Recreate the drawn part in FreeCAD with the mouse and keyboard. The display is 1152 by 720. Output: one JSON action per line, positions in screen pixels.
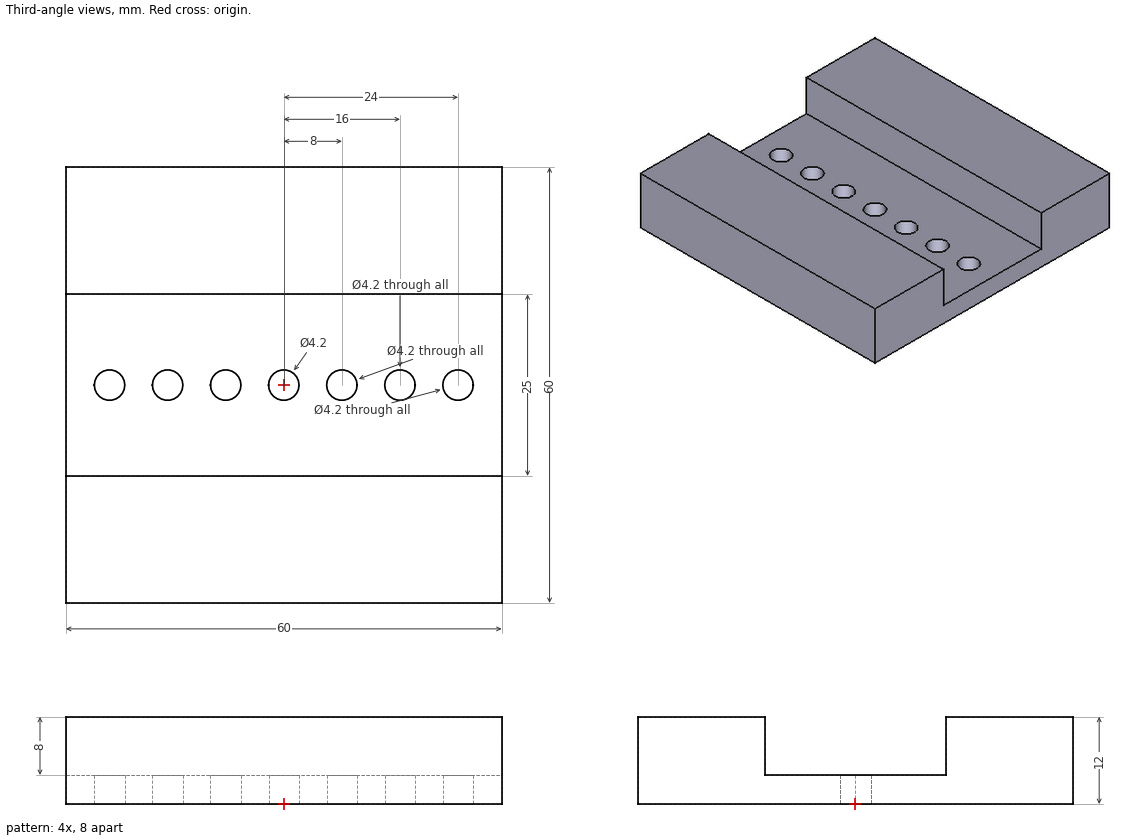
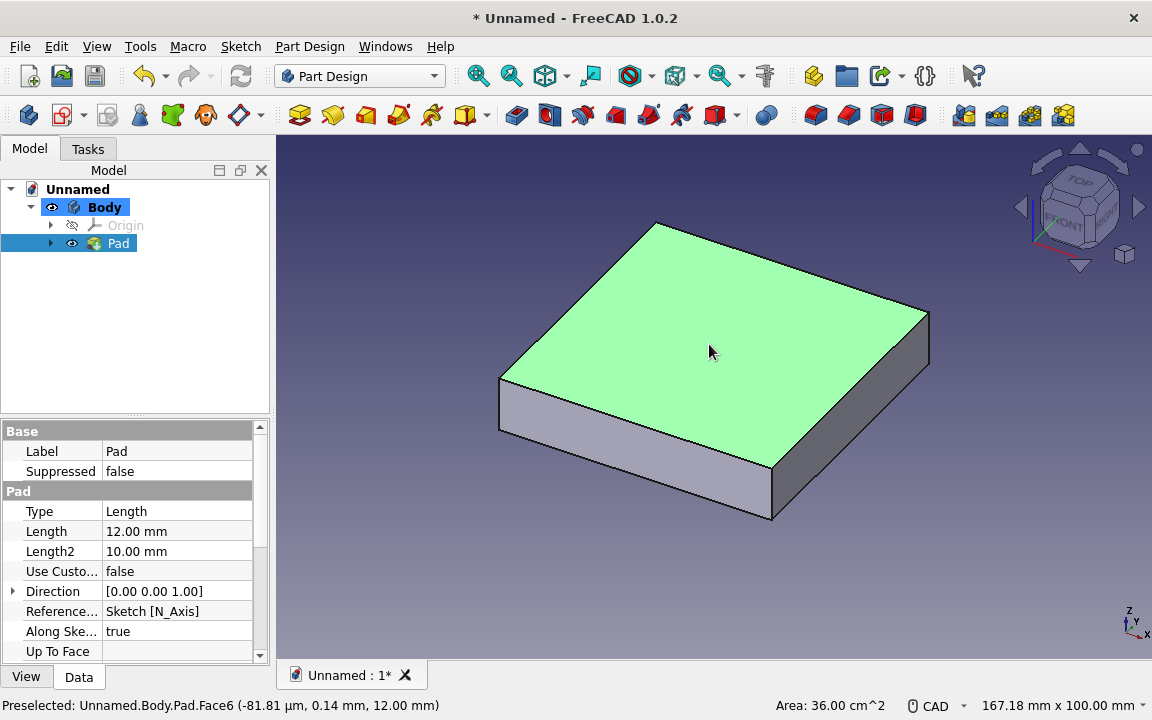
{"action": "left_click", "coordinate": [62, 116]}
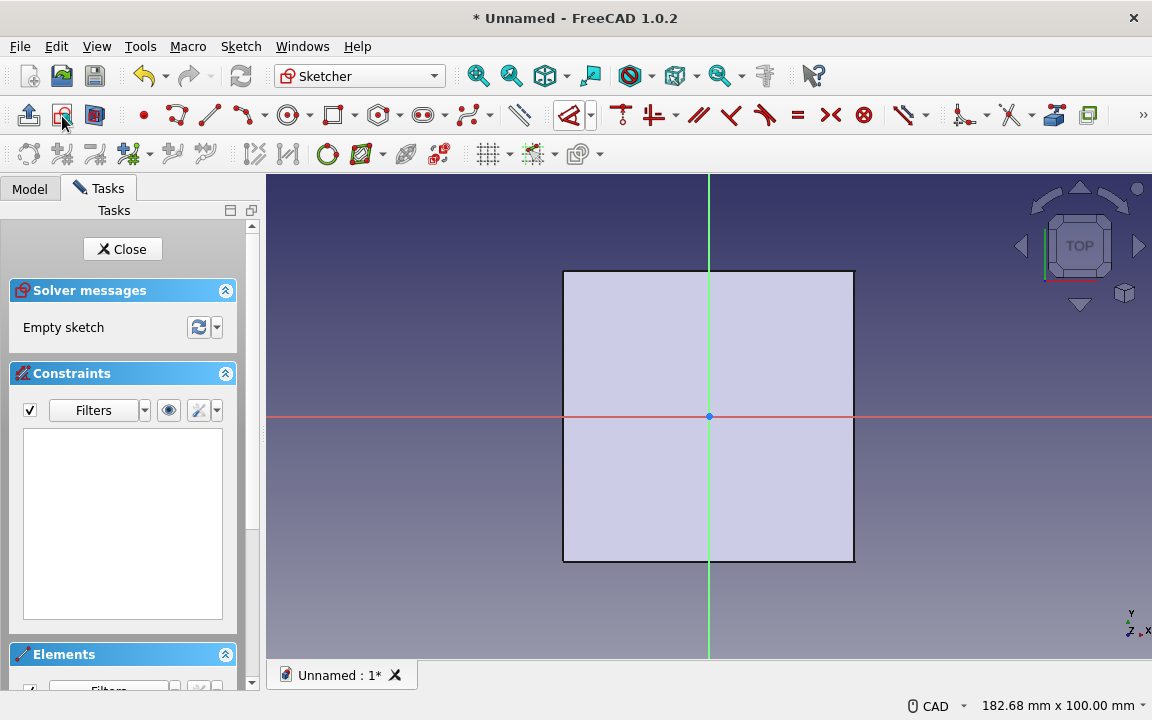
{"action": "scroll", "coordinate": [792, 416], "scroll_direction": "up", "scroll_amount": 3}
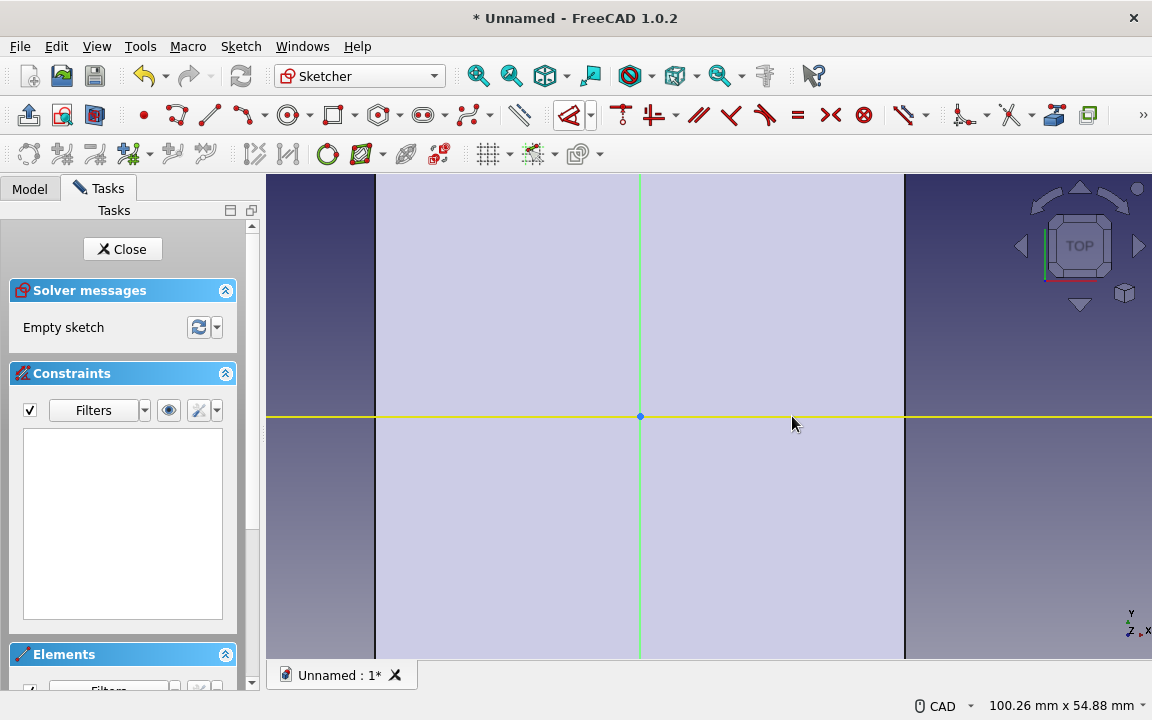
{"action": "left_click", "coordinate": [354, 116]}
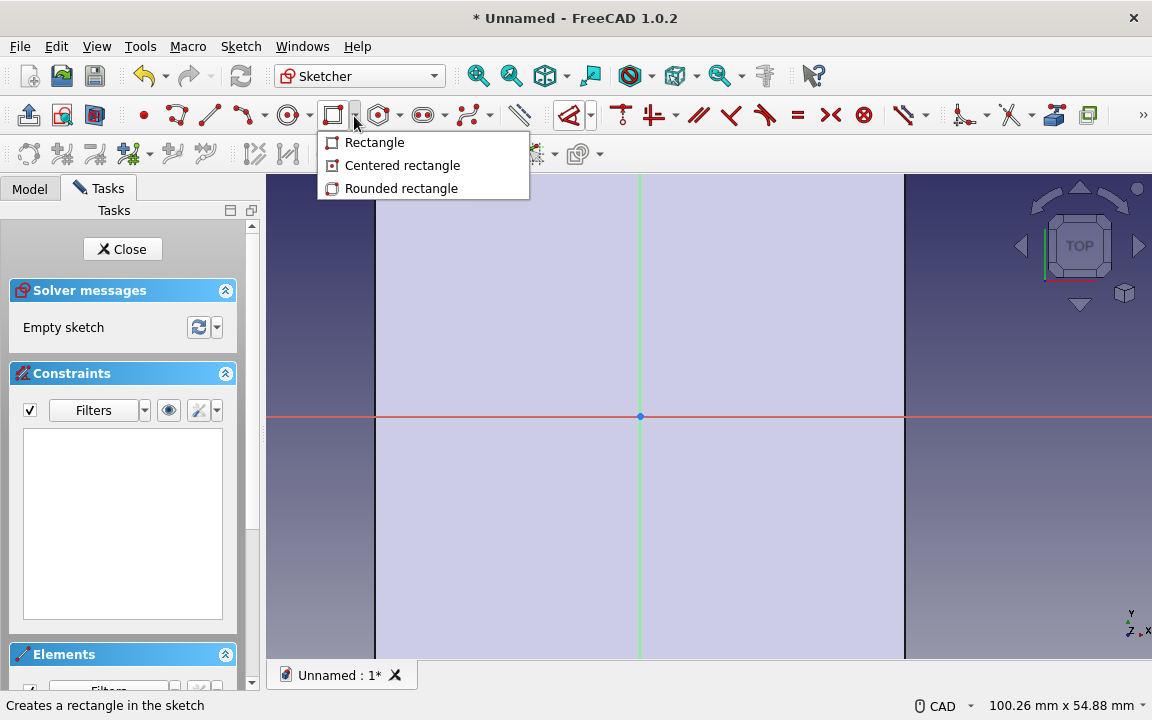
{"action": "left_click", "coordinate": [424, 166]}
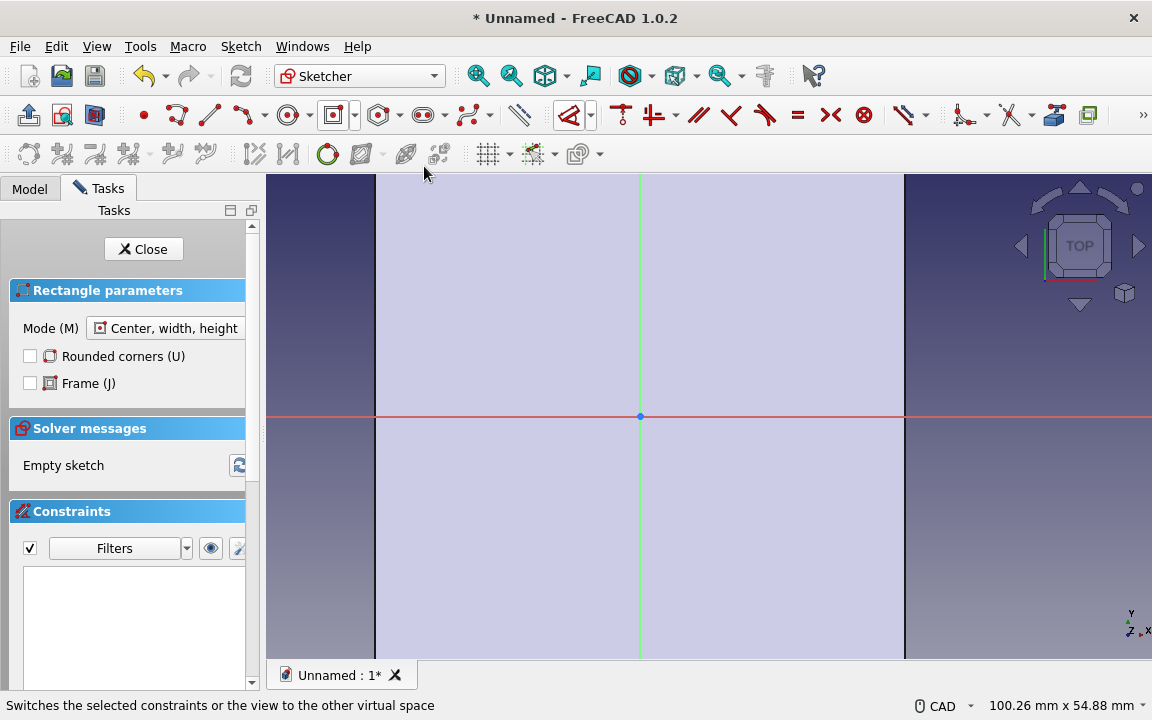
{"action": "left_click", "coordinate": [640, 416]}
{"action": "mouse_move", "coordinate": [905, 306]}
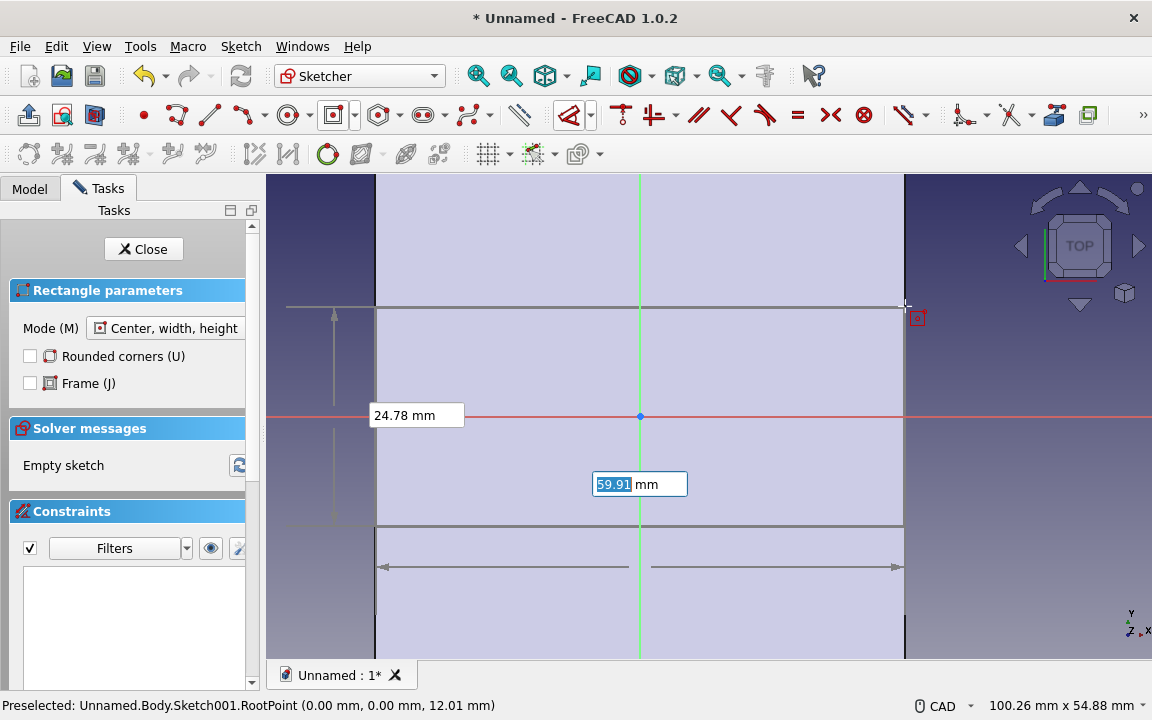
{"action": "type", "text": "60"}
{"action": "key", "text": "Tab"}
{"action": "type", "text": "25"}
{"action": "key", "text": "Return"}
{"action": "key", "text": "Escape"}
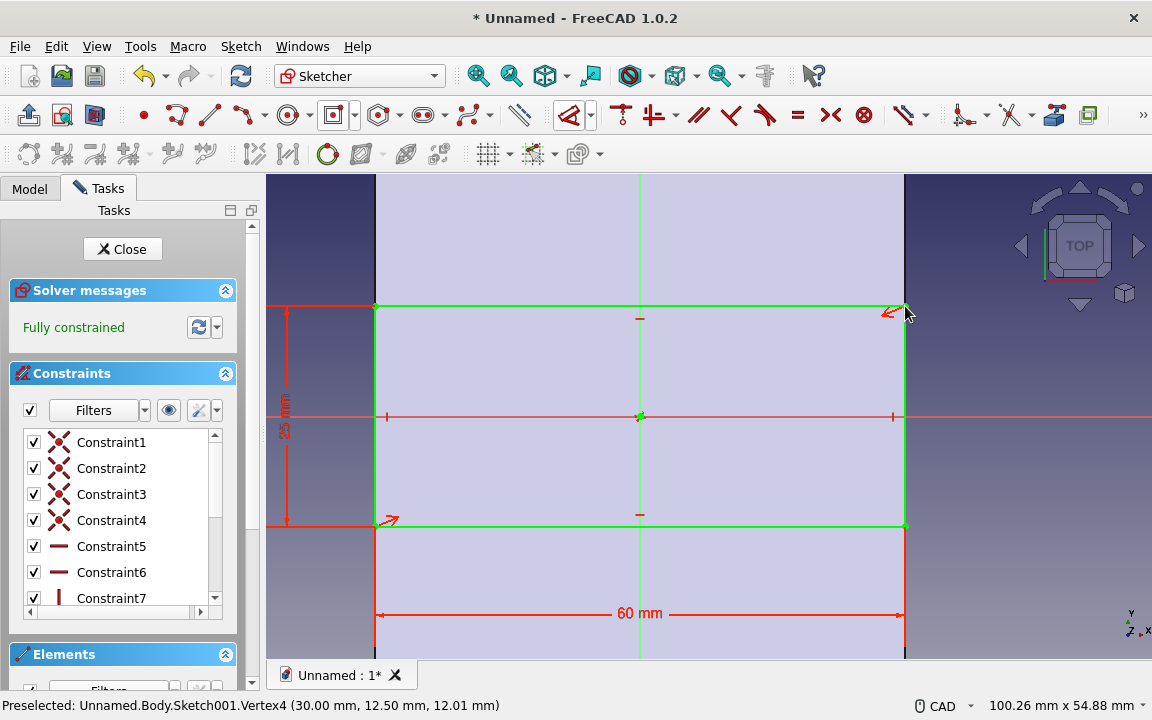
{"action": "left_click", "coordinate": [123, 249]}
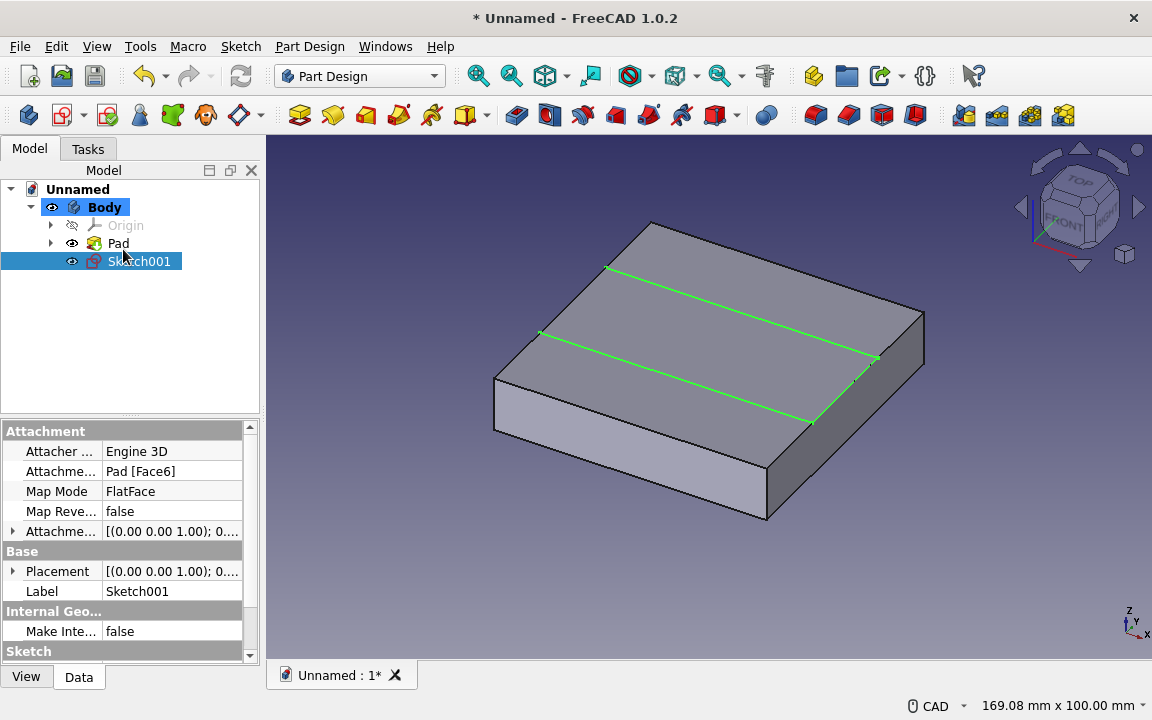
{"action": "left_click", "coordinate": [517, 116]}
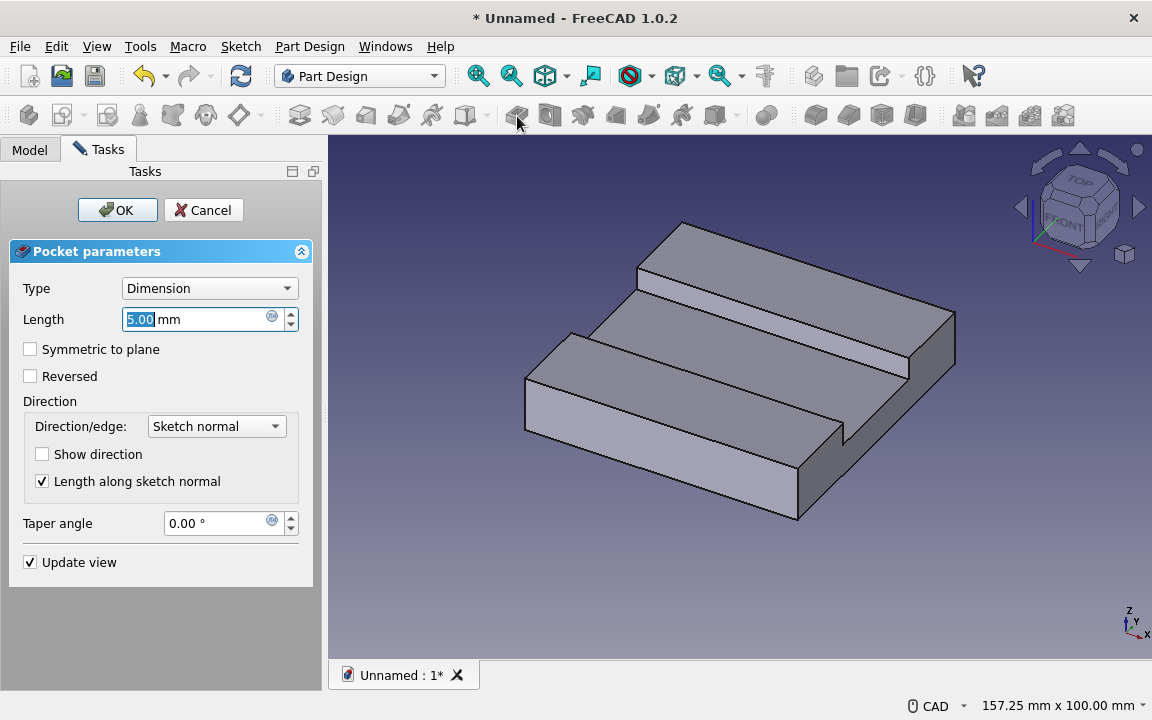
{"action": "type", "text": "8"}
{"action": "key", "text": "Tab"}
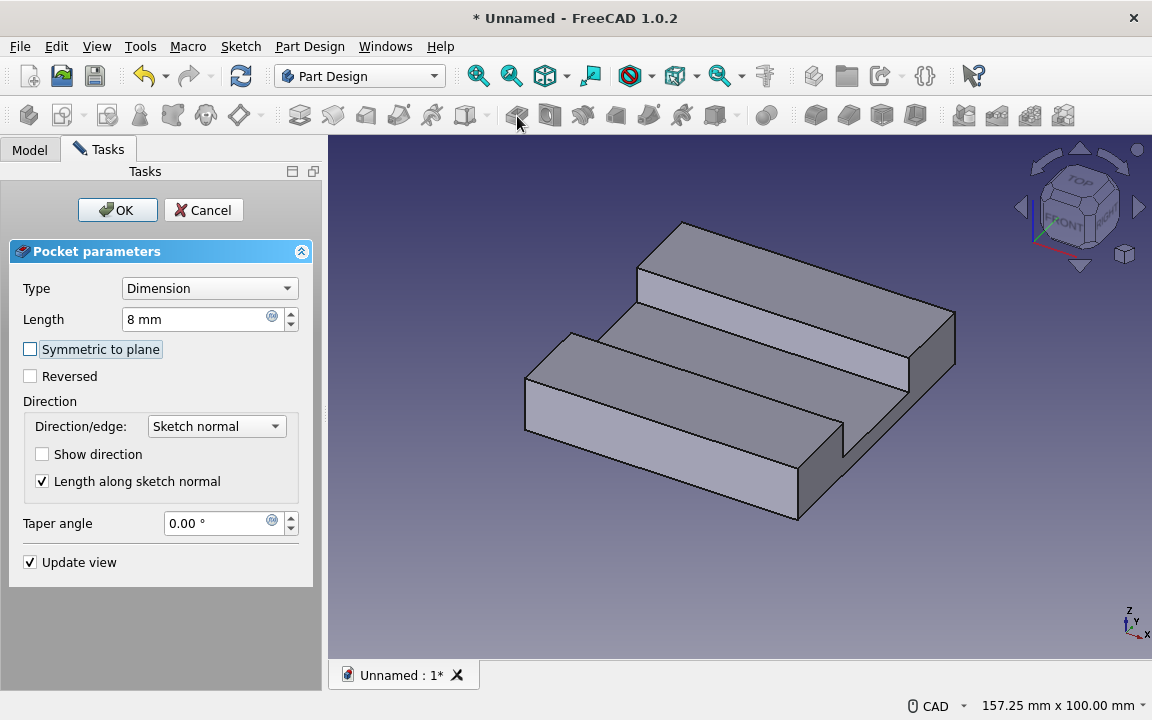
{"action": "left_click", "coordinate": [118, 210]}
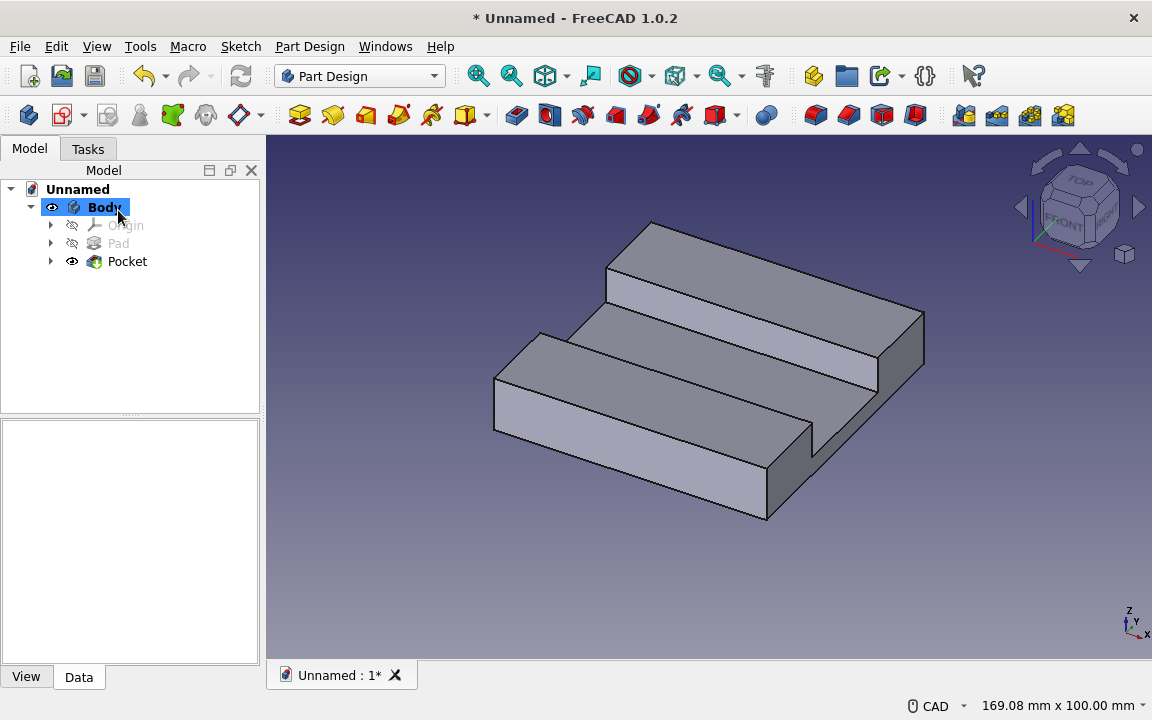
{"action": "key", "text": "0"}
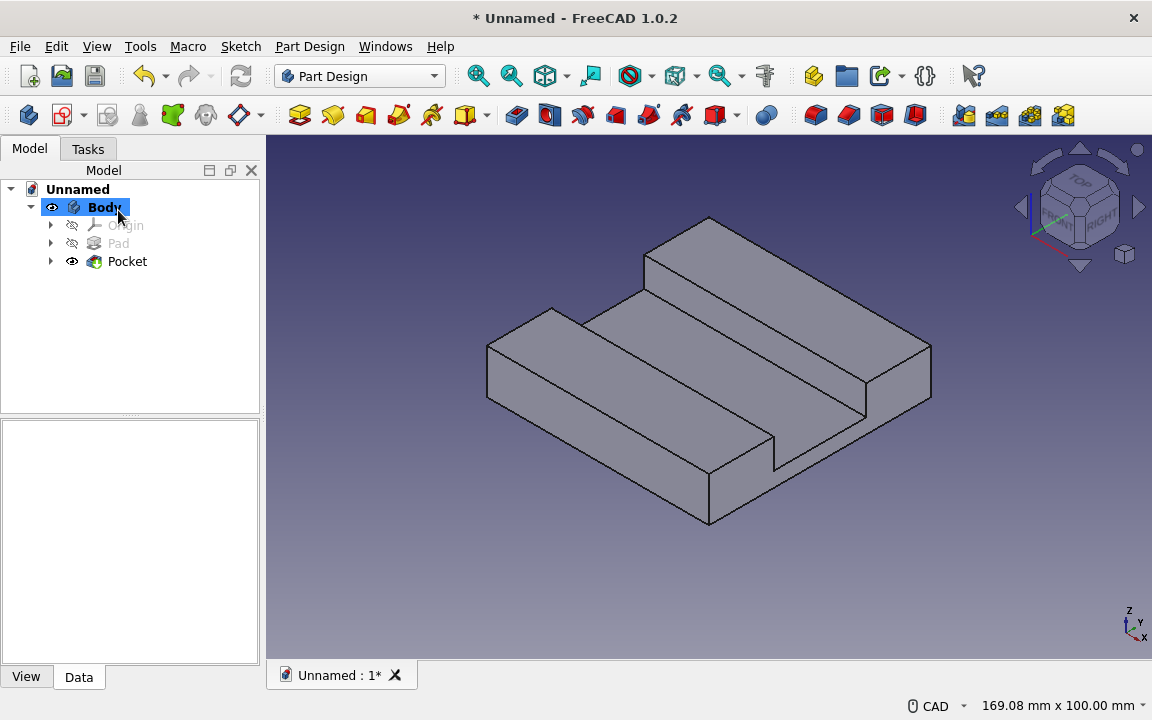
{"action": "left_click", "coordinate": [773, 416]}